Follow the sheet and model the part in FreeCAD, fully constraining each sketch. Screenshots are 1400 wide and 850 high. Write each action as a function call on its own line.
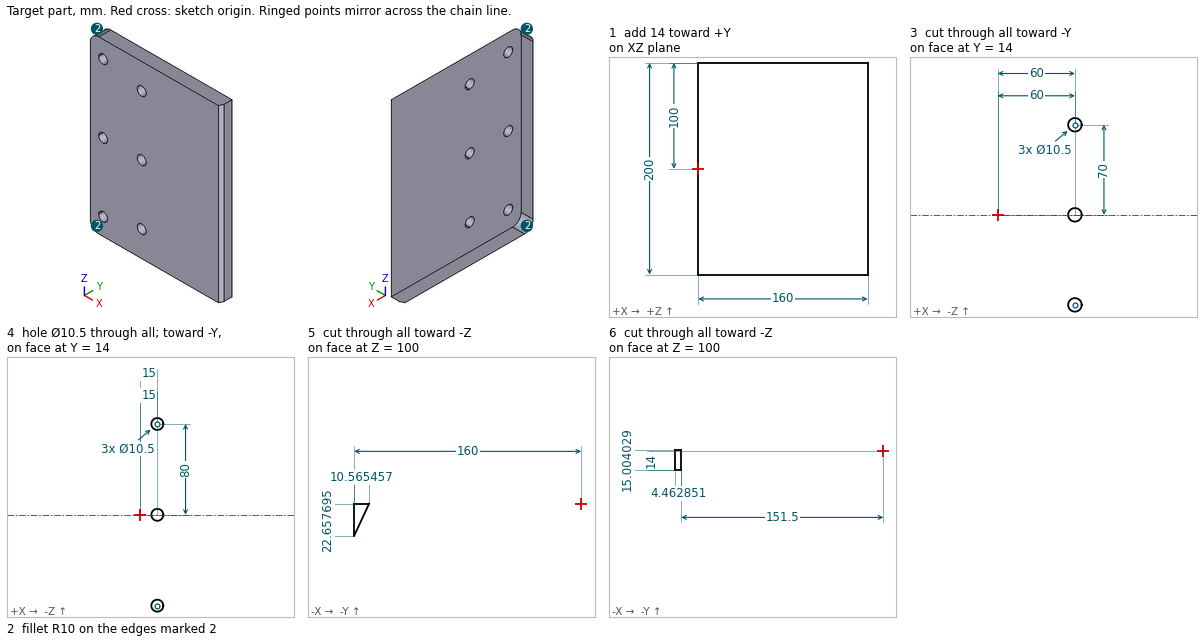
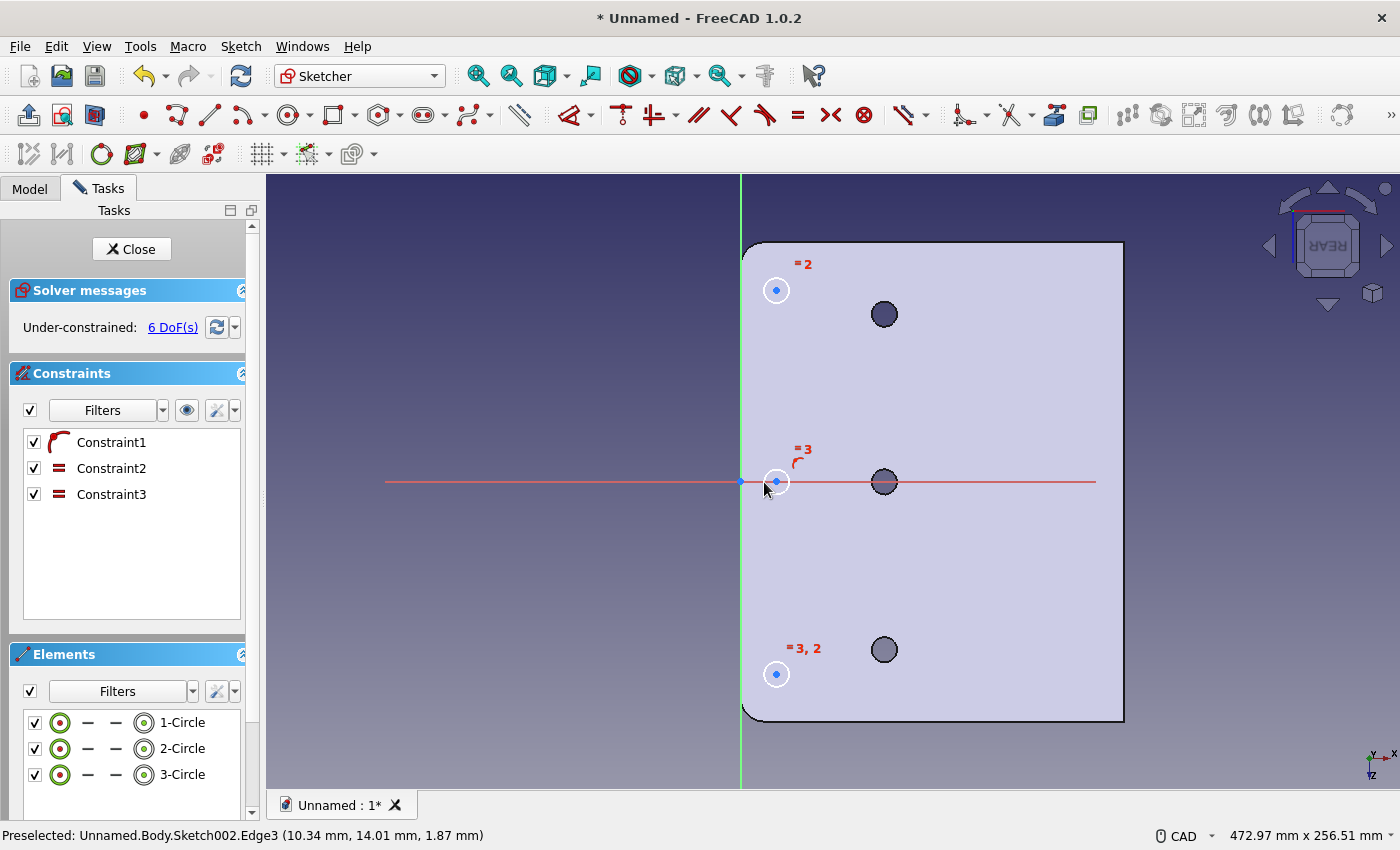
click(777, 291)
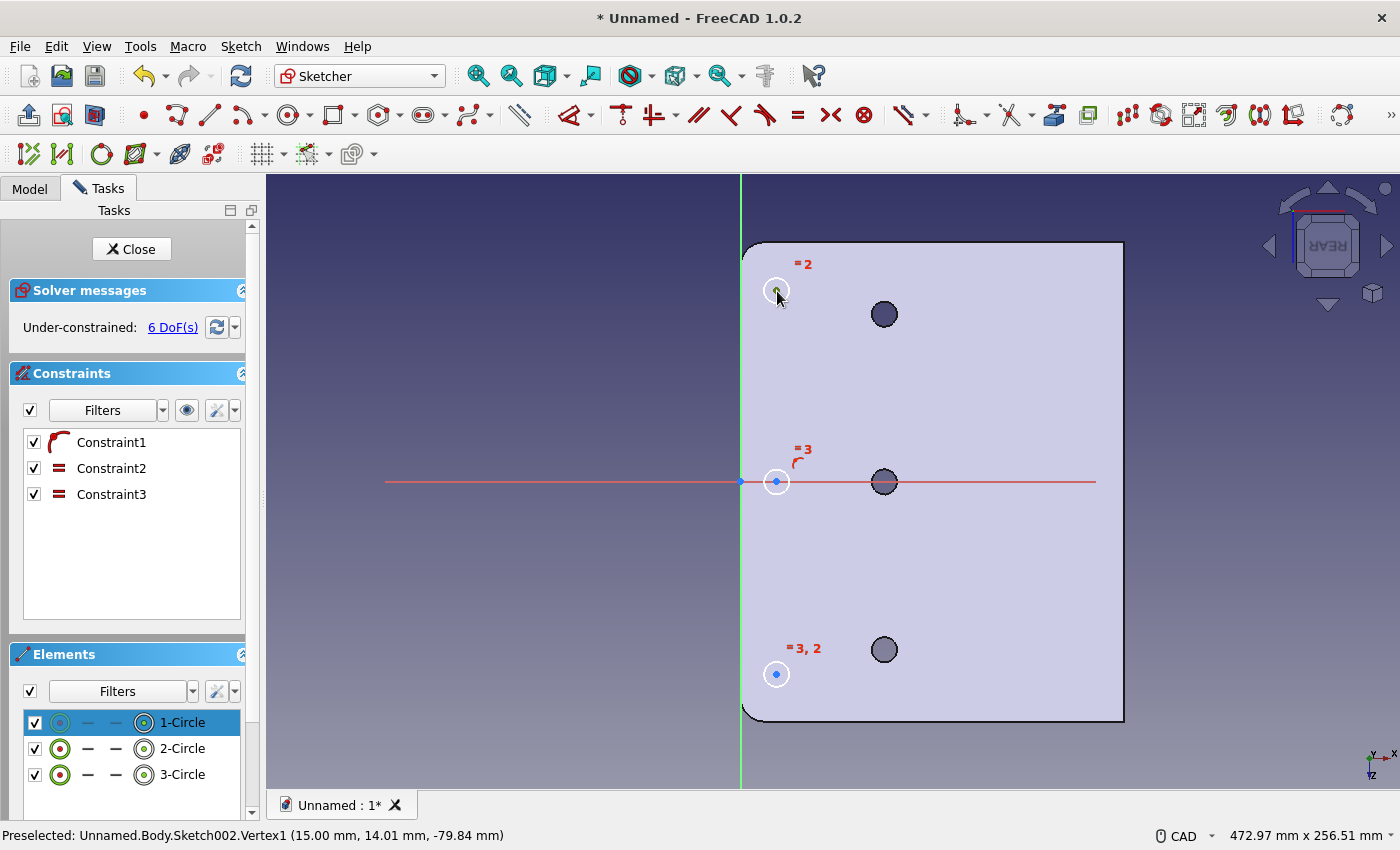
click(777, 674)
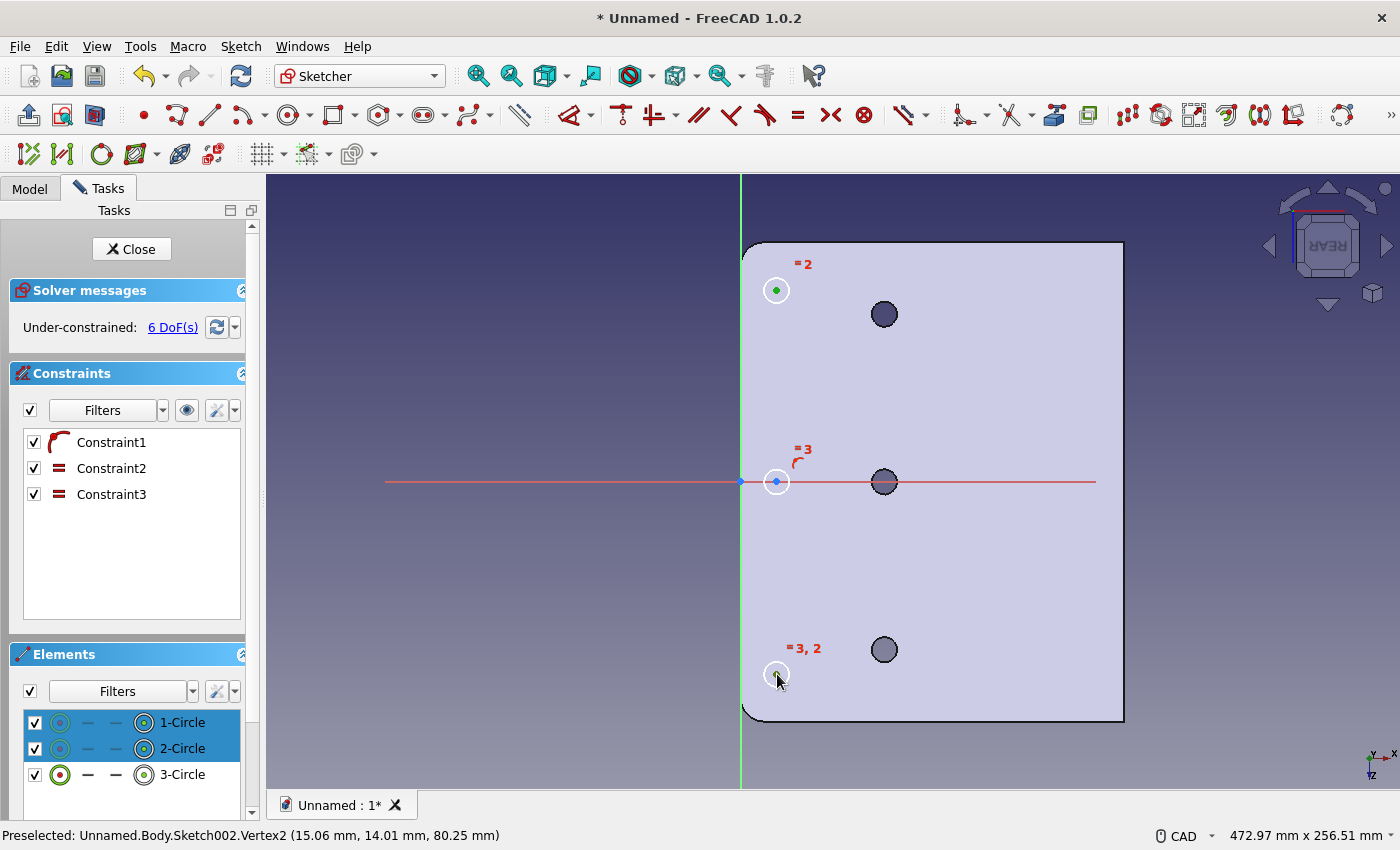
click(428, 482)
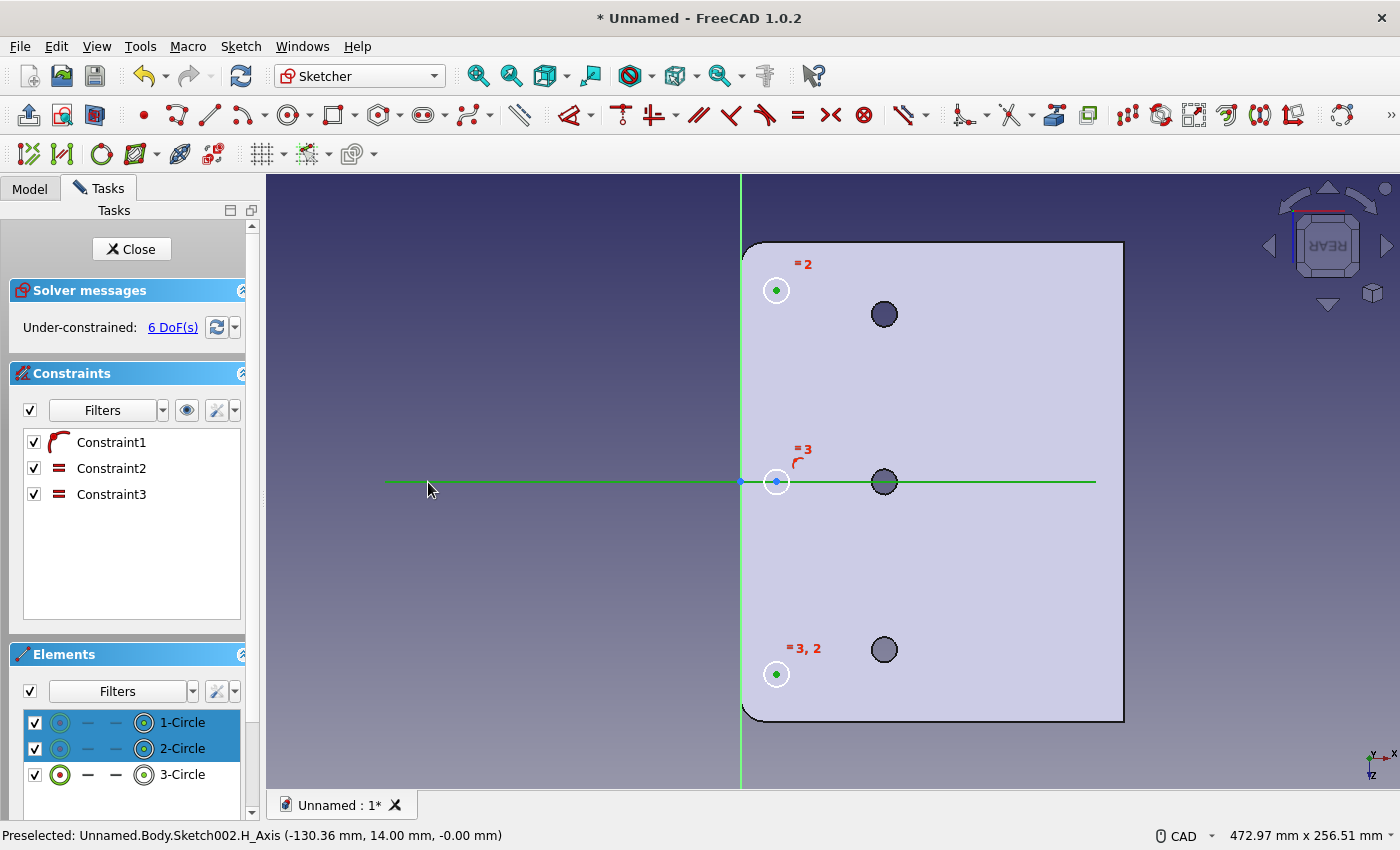
key(s)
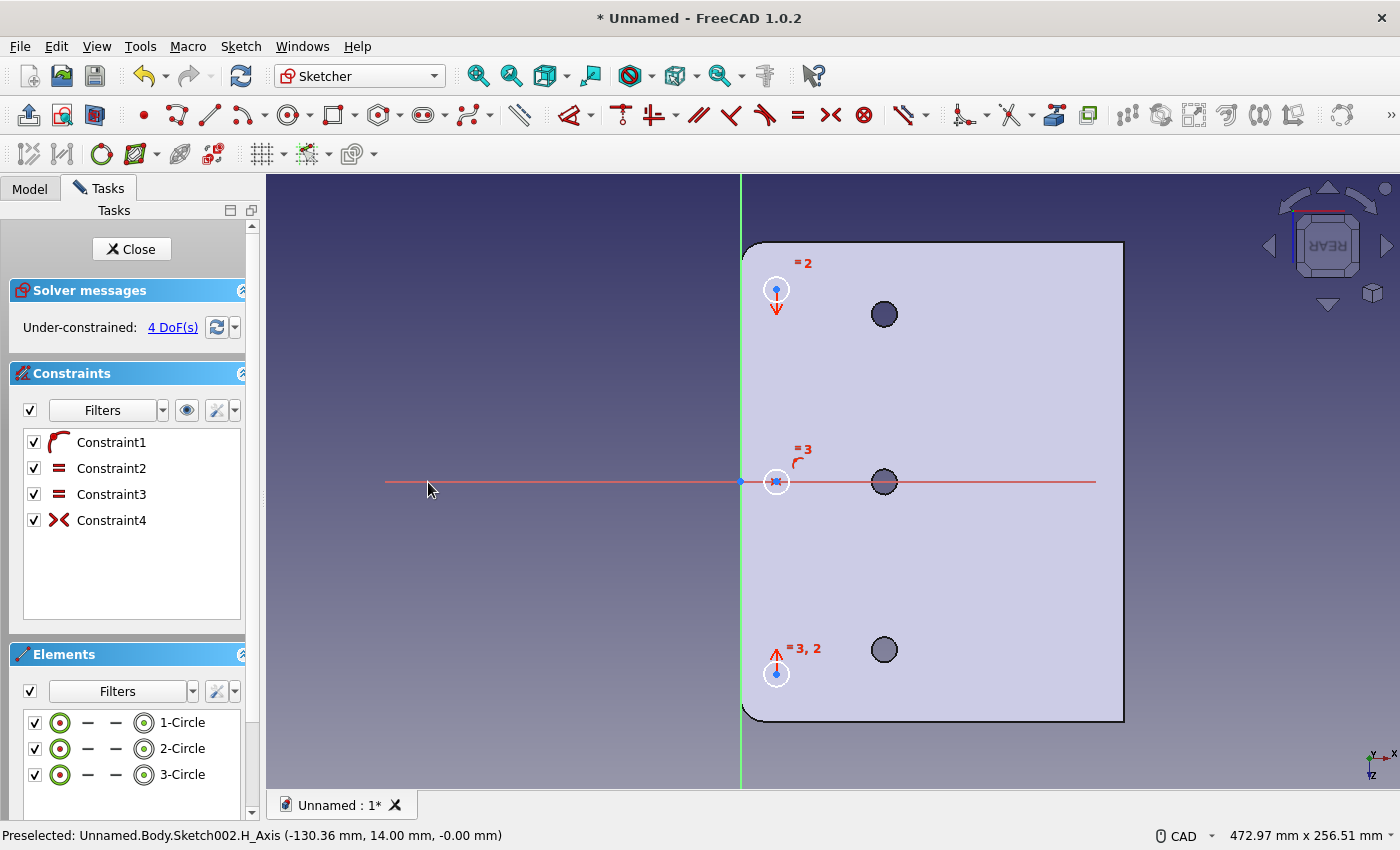
click(568, 116)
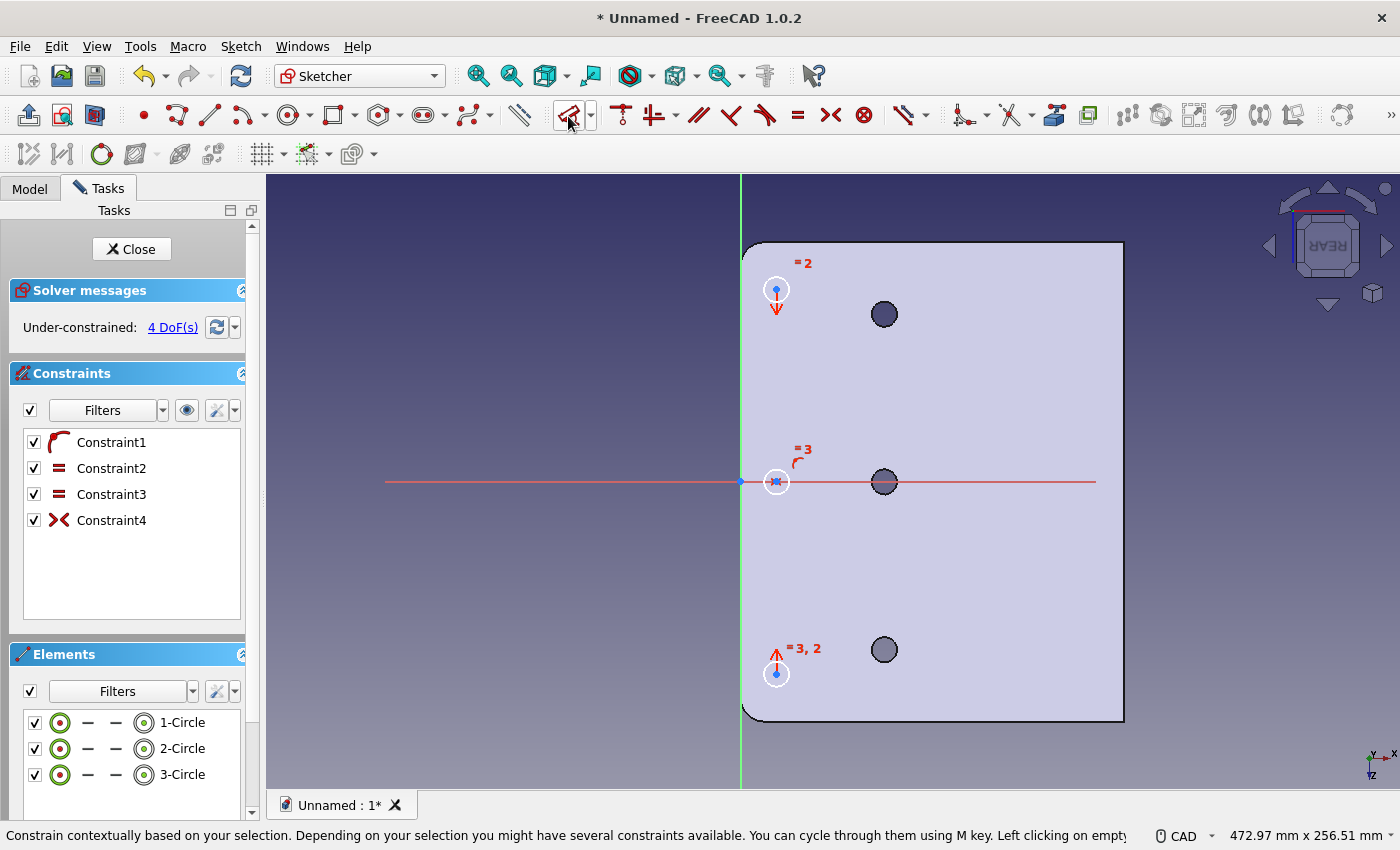
scroll(785, 281, up, 3)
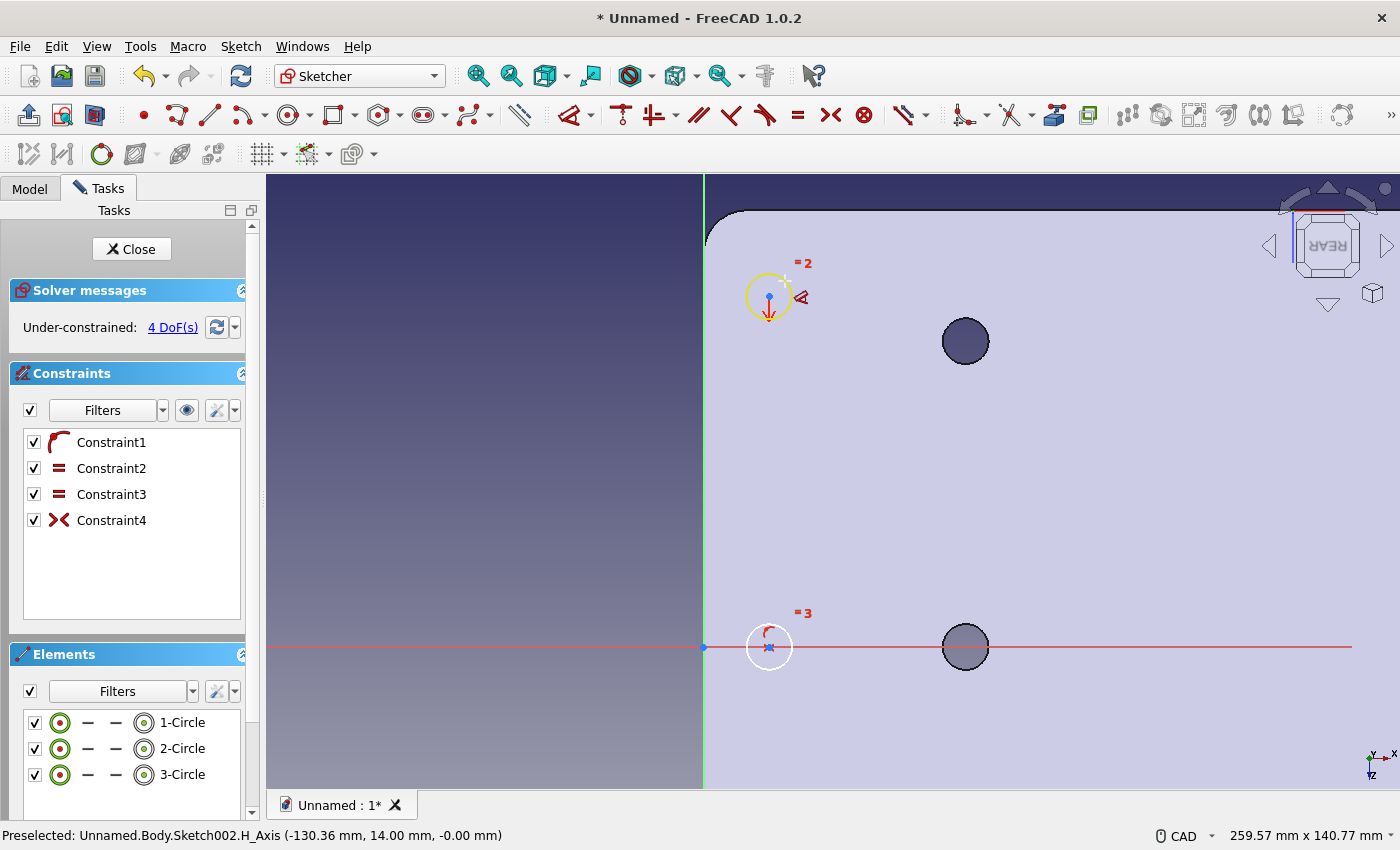
click(785, 281)
click(808, 258)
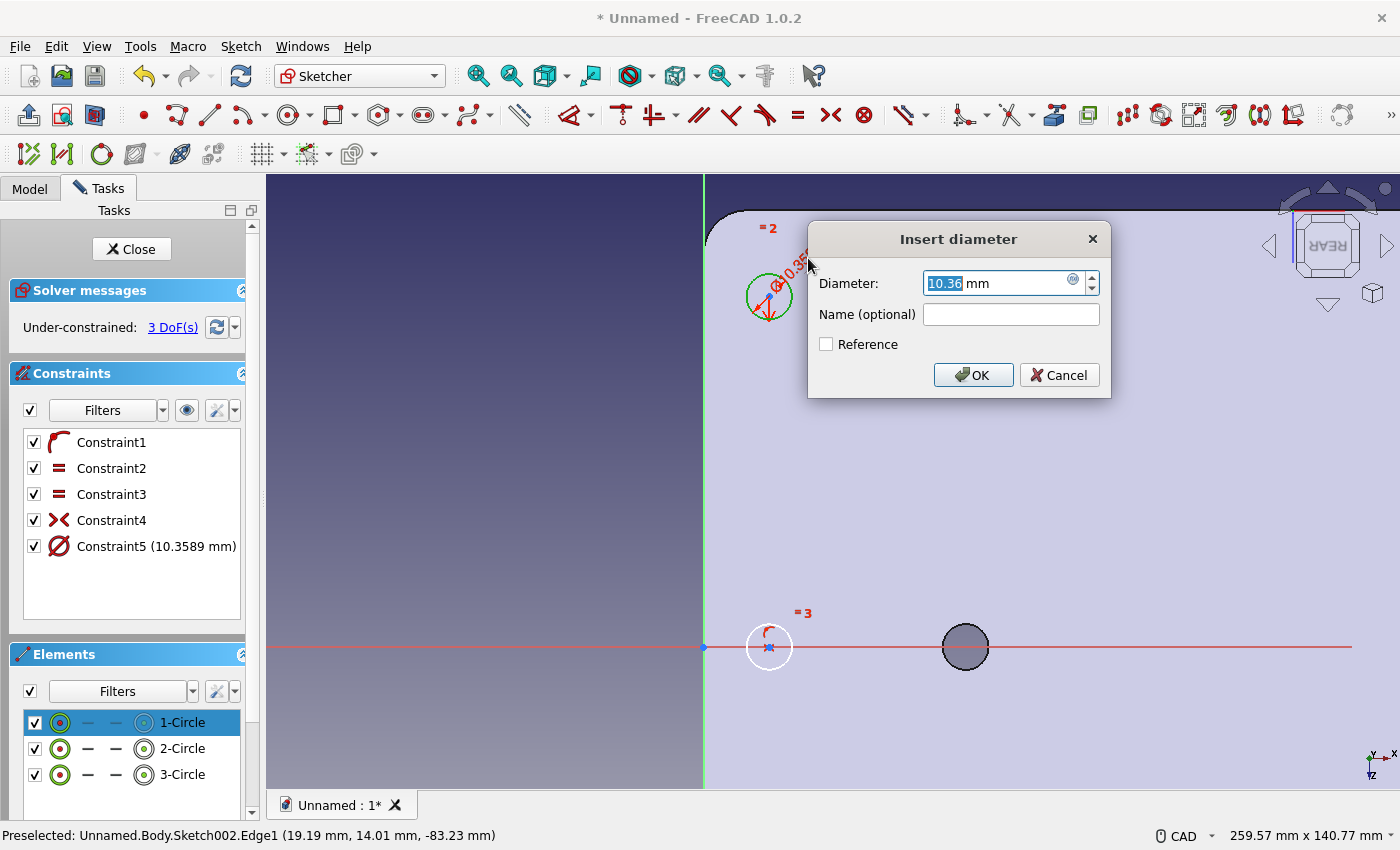
text(10.5)
key(Return)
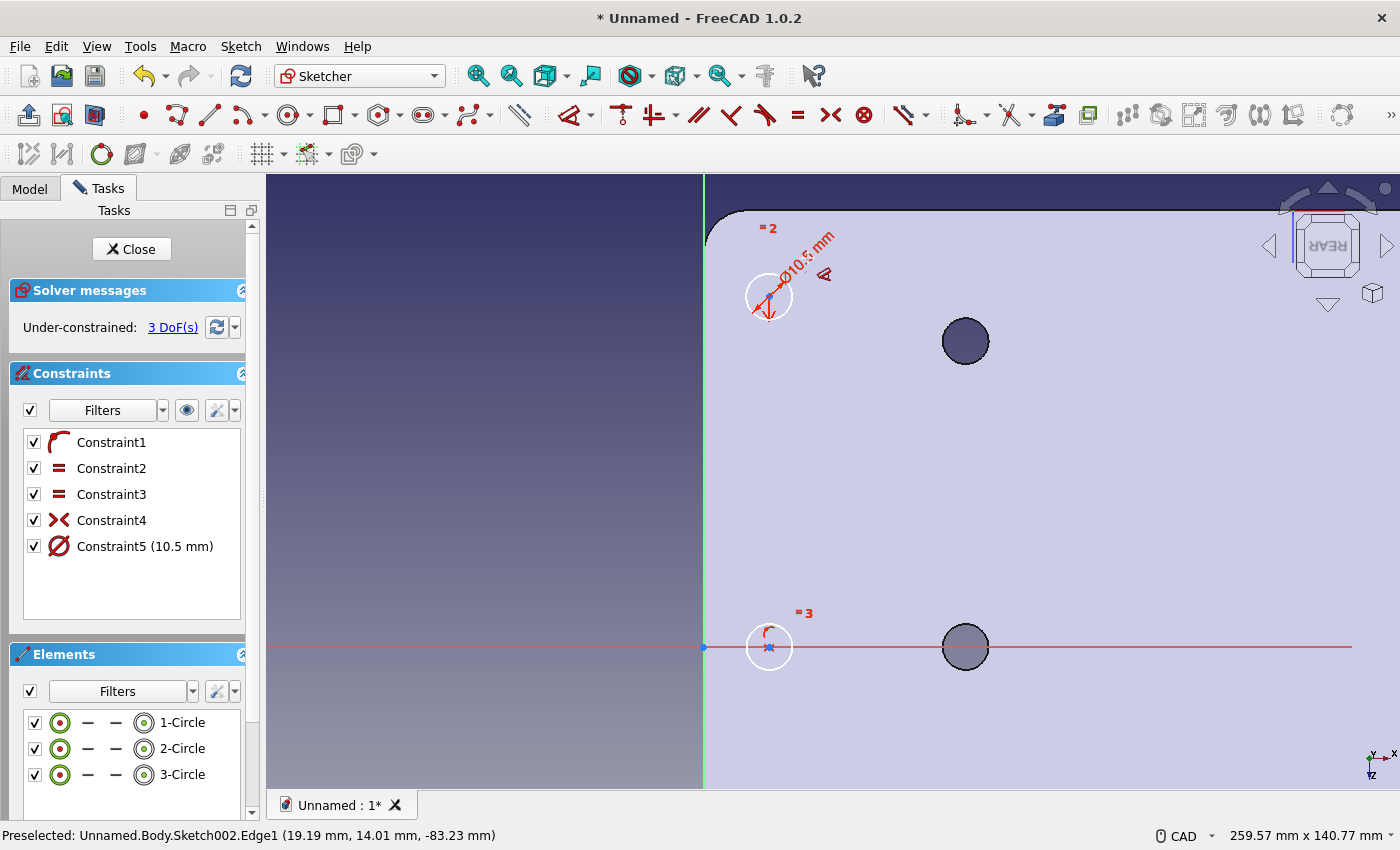
click(769, 297)
click(736, 263)